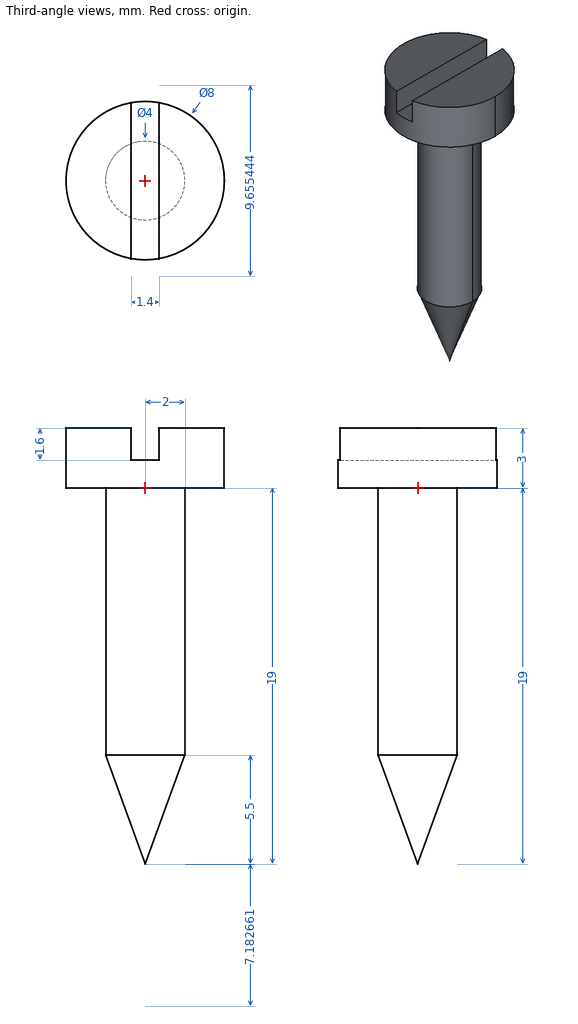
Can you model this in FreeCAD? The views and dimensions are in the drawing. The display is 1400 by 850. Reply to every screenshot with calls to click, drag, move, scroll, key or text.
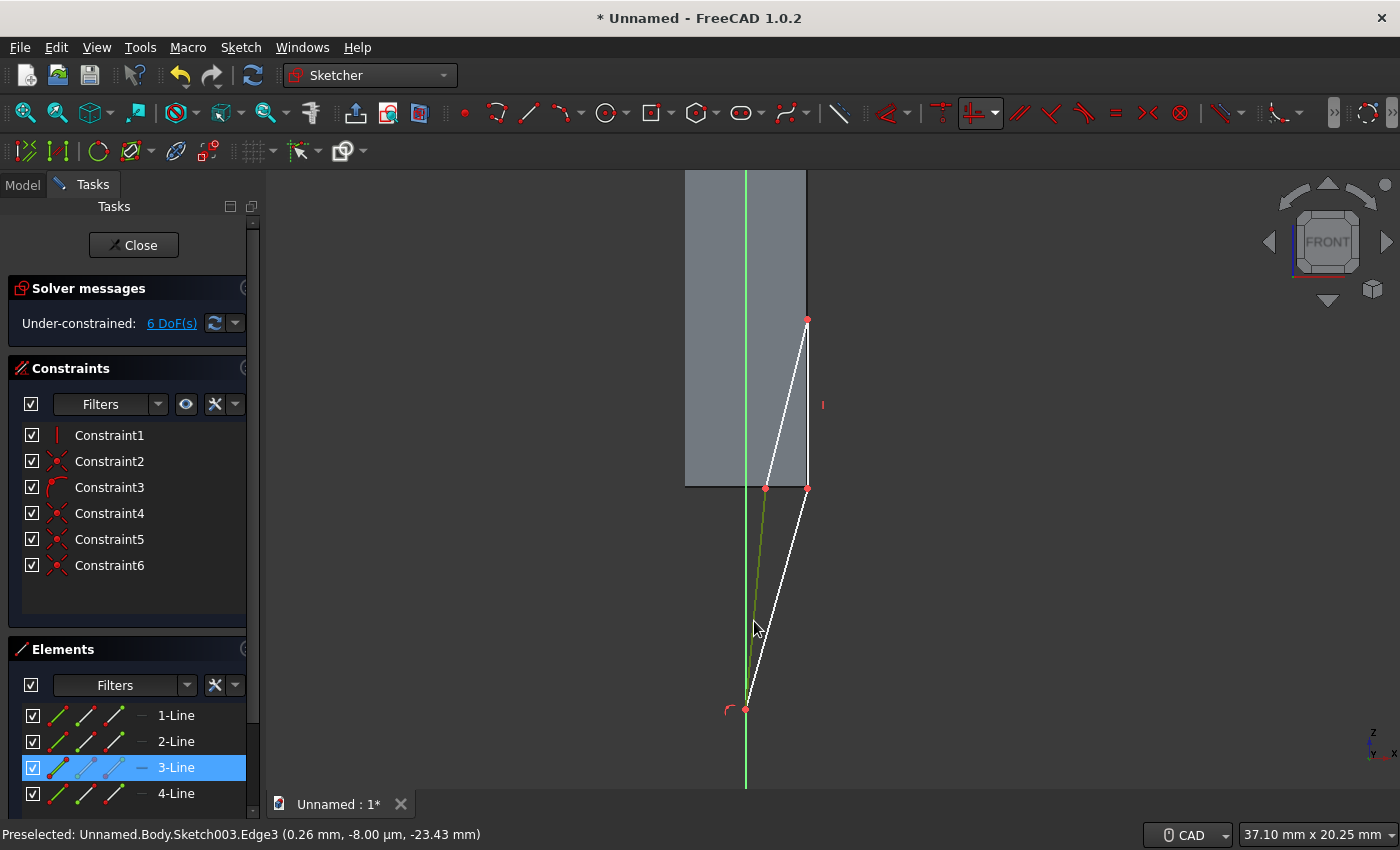
key(v)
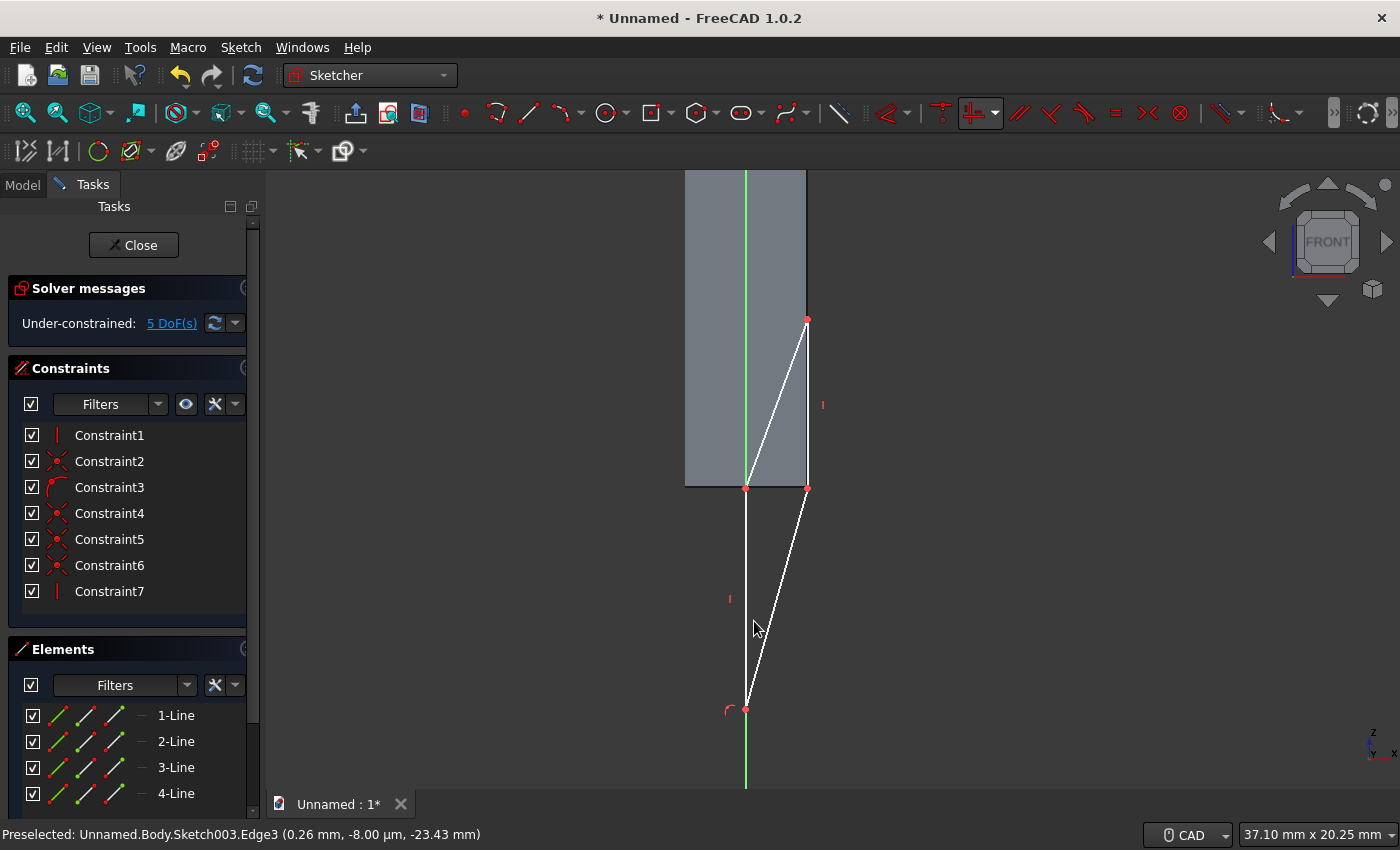
key(d)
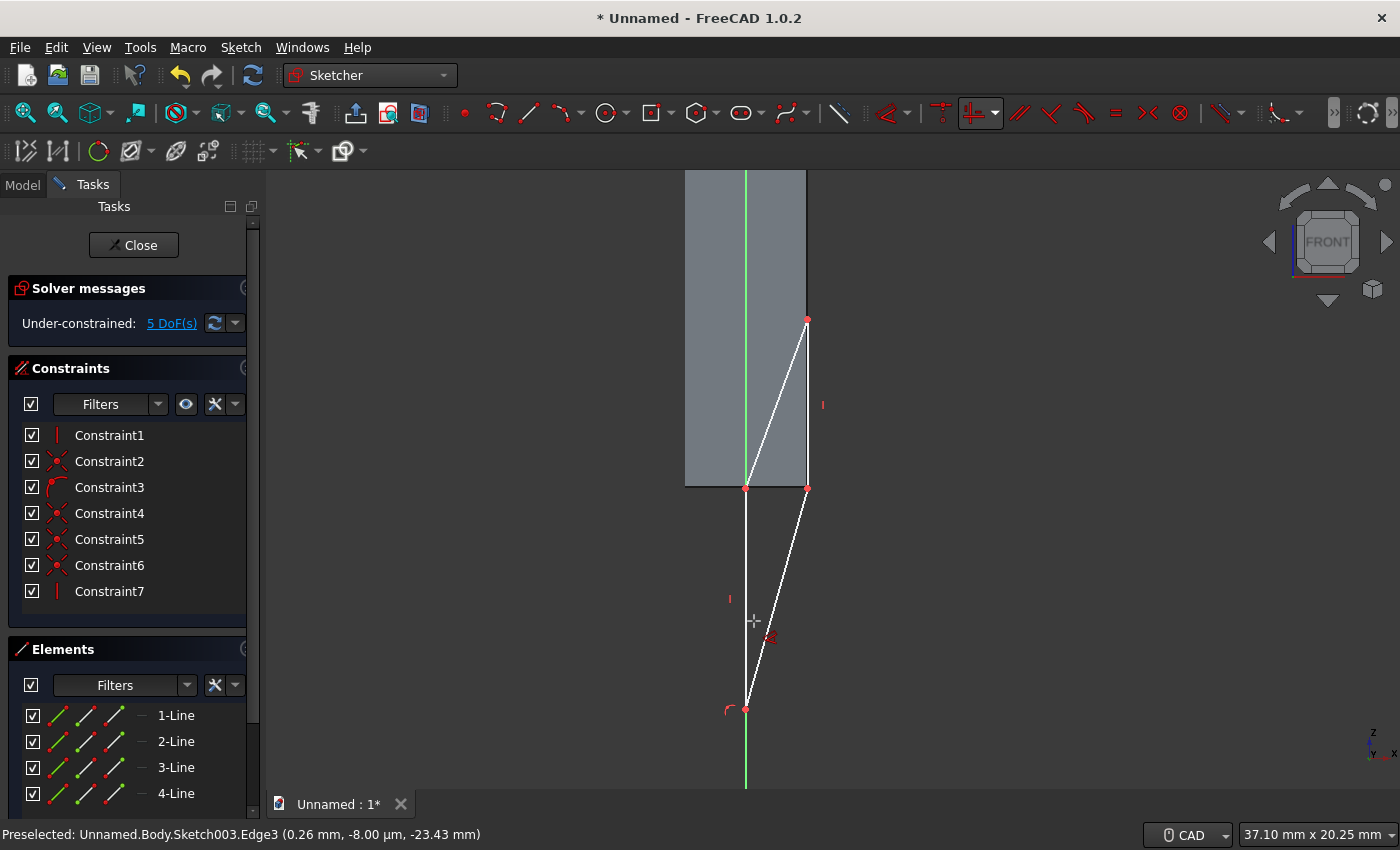
click(808, 320)
click(777, 354)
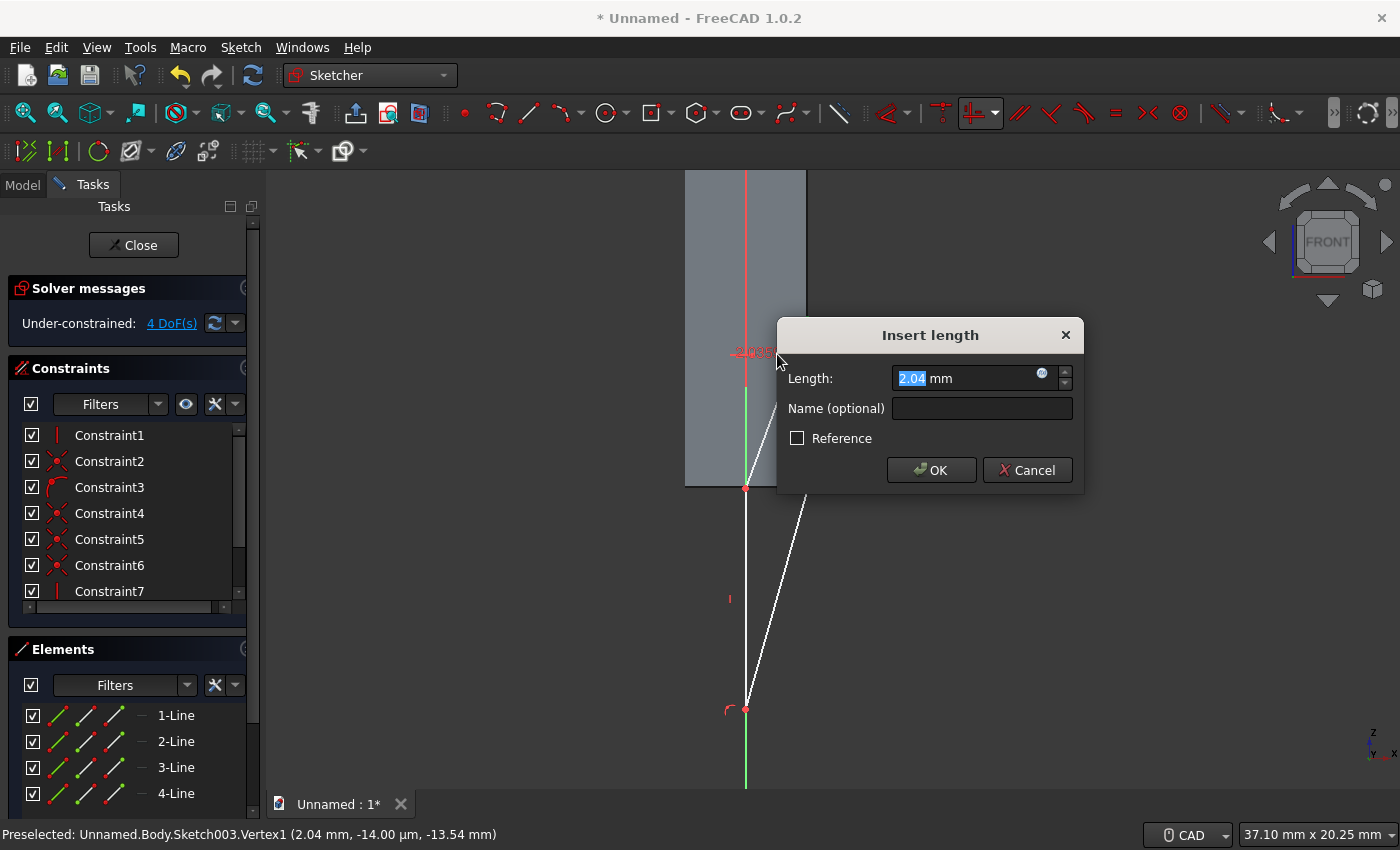
text(2)
key(Return)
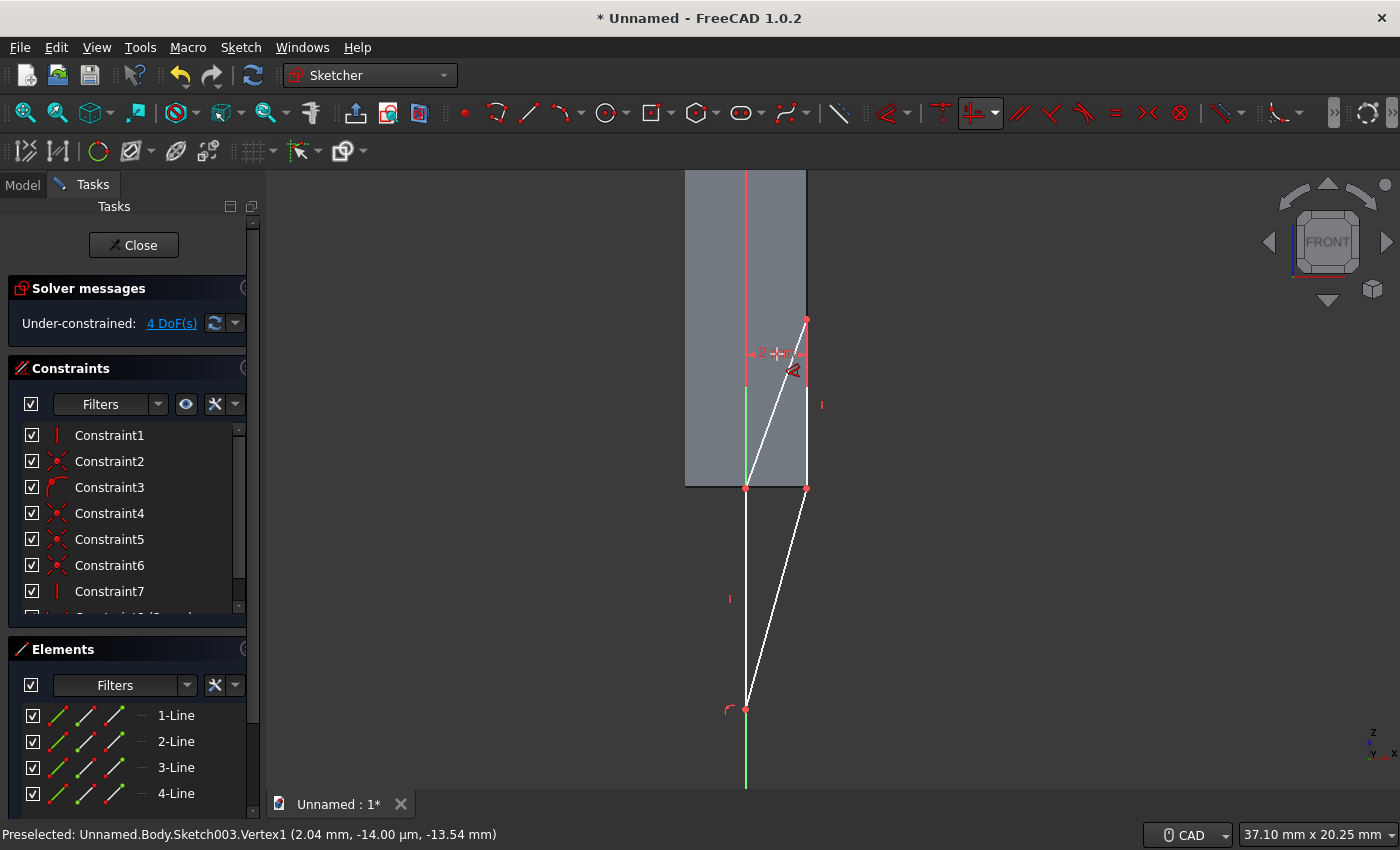
click(807, 370)
click(841, 404)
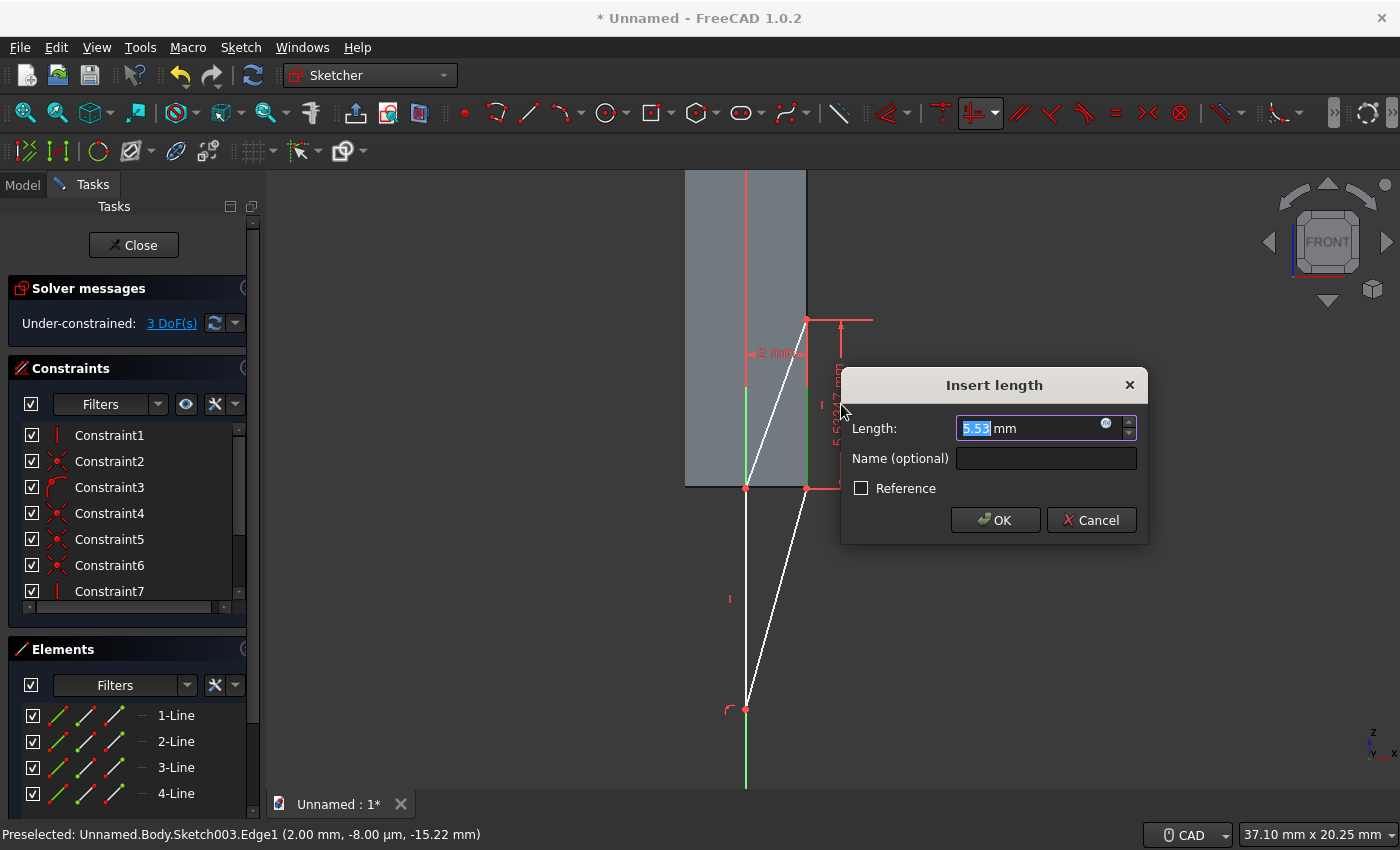
text(5.5)
key(Return)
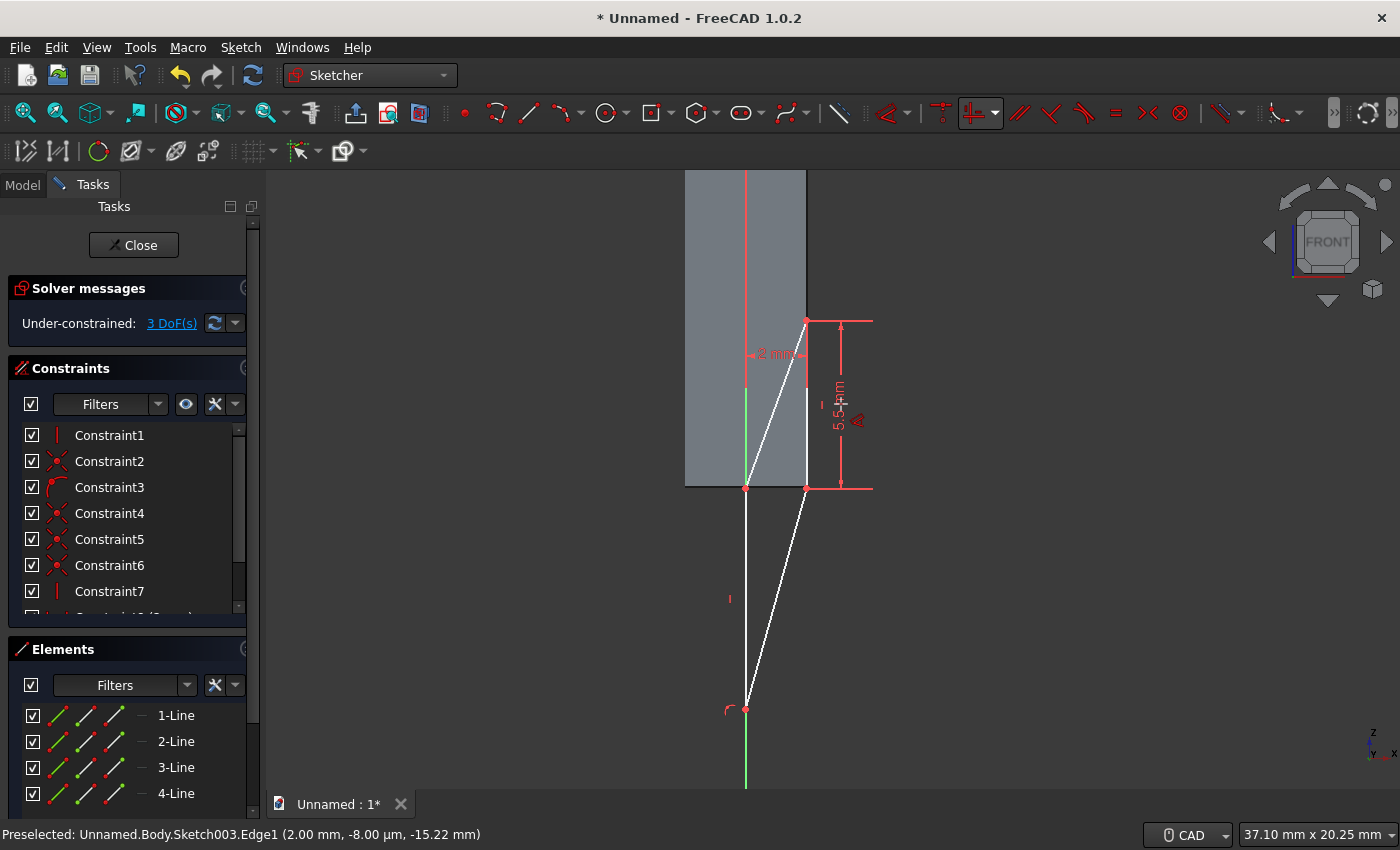
click(807, 489)
click(712, 277)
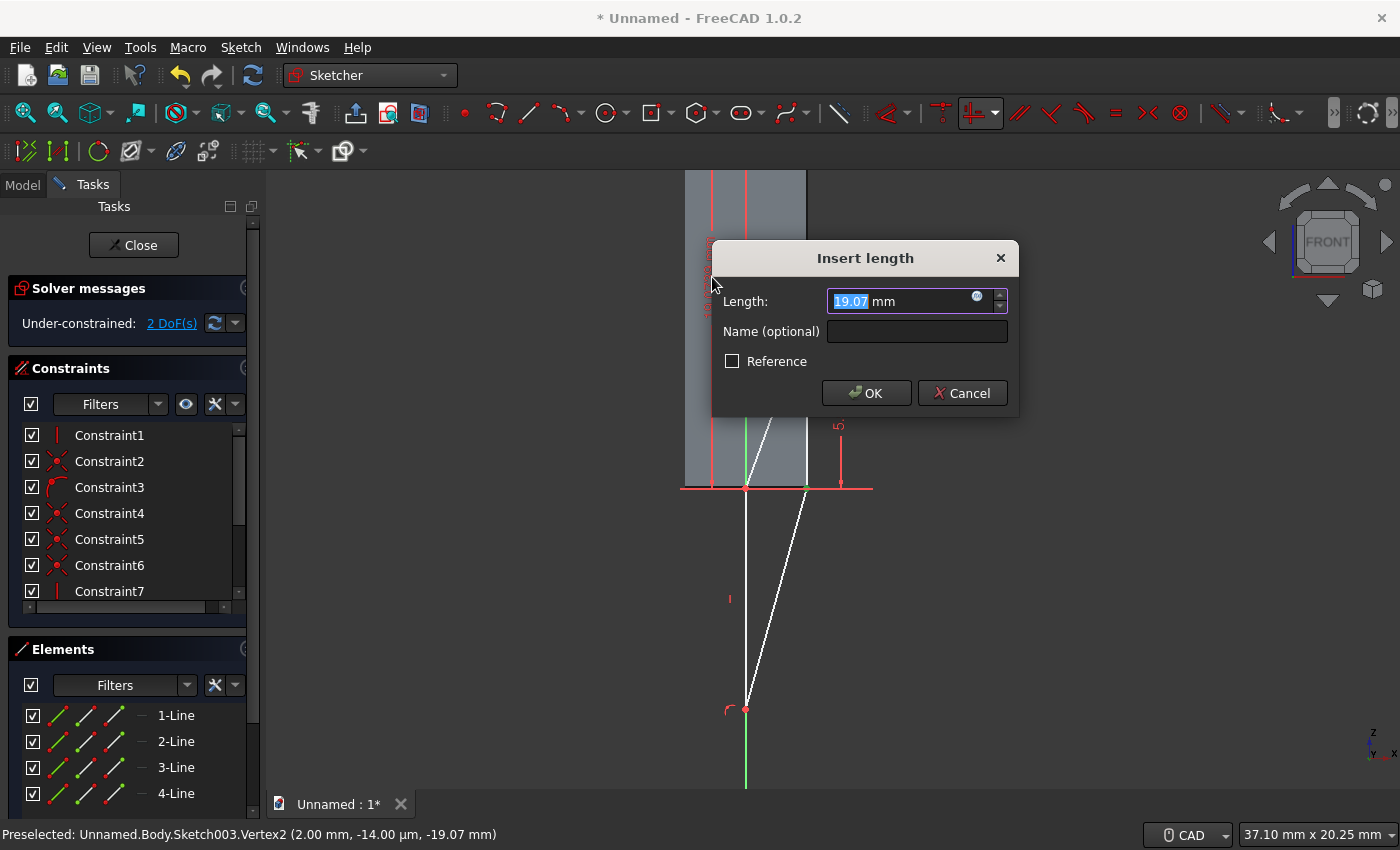
text(19)
key(Return)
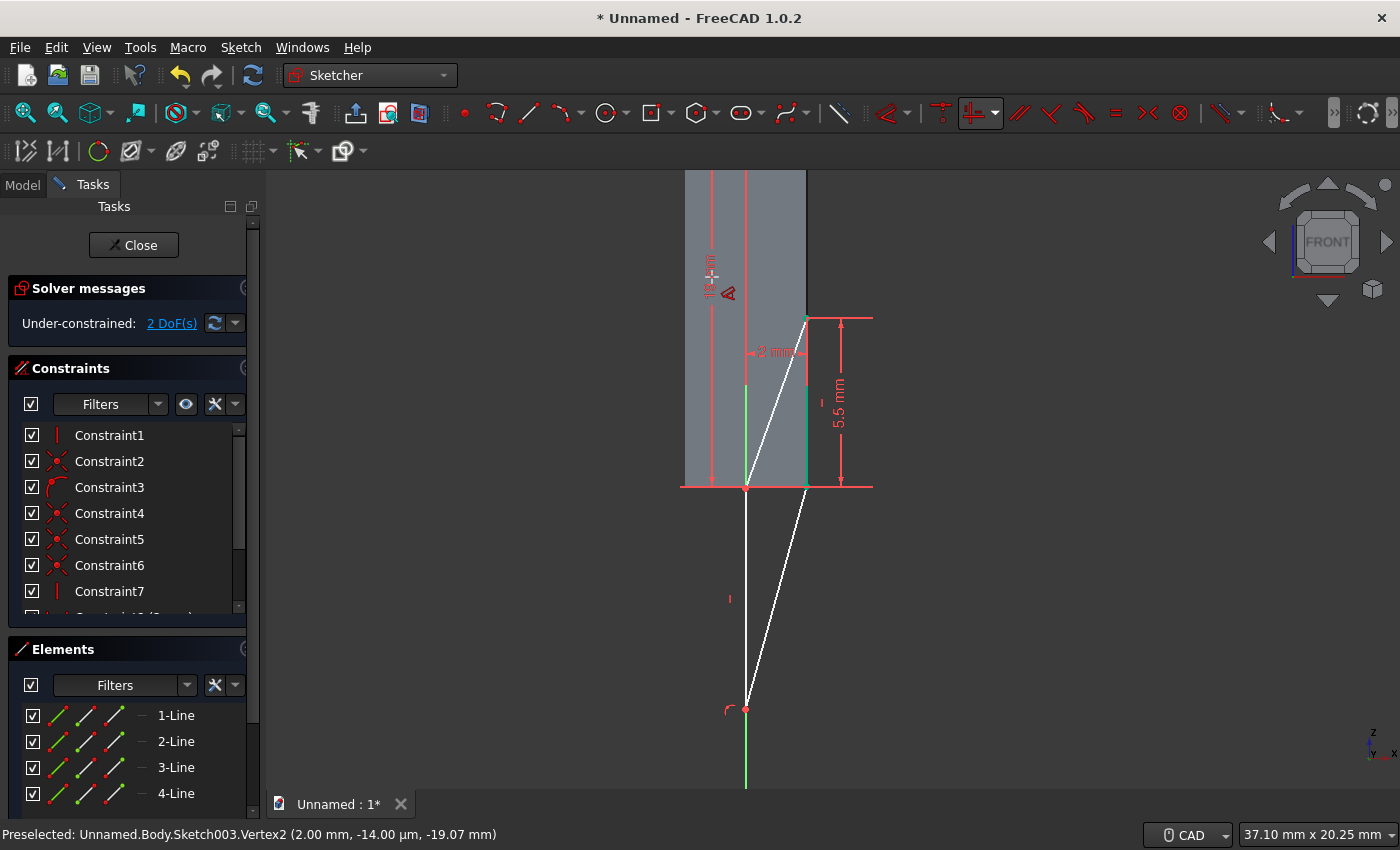
click(746, 489)
click(712, 410)